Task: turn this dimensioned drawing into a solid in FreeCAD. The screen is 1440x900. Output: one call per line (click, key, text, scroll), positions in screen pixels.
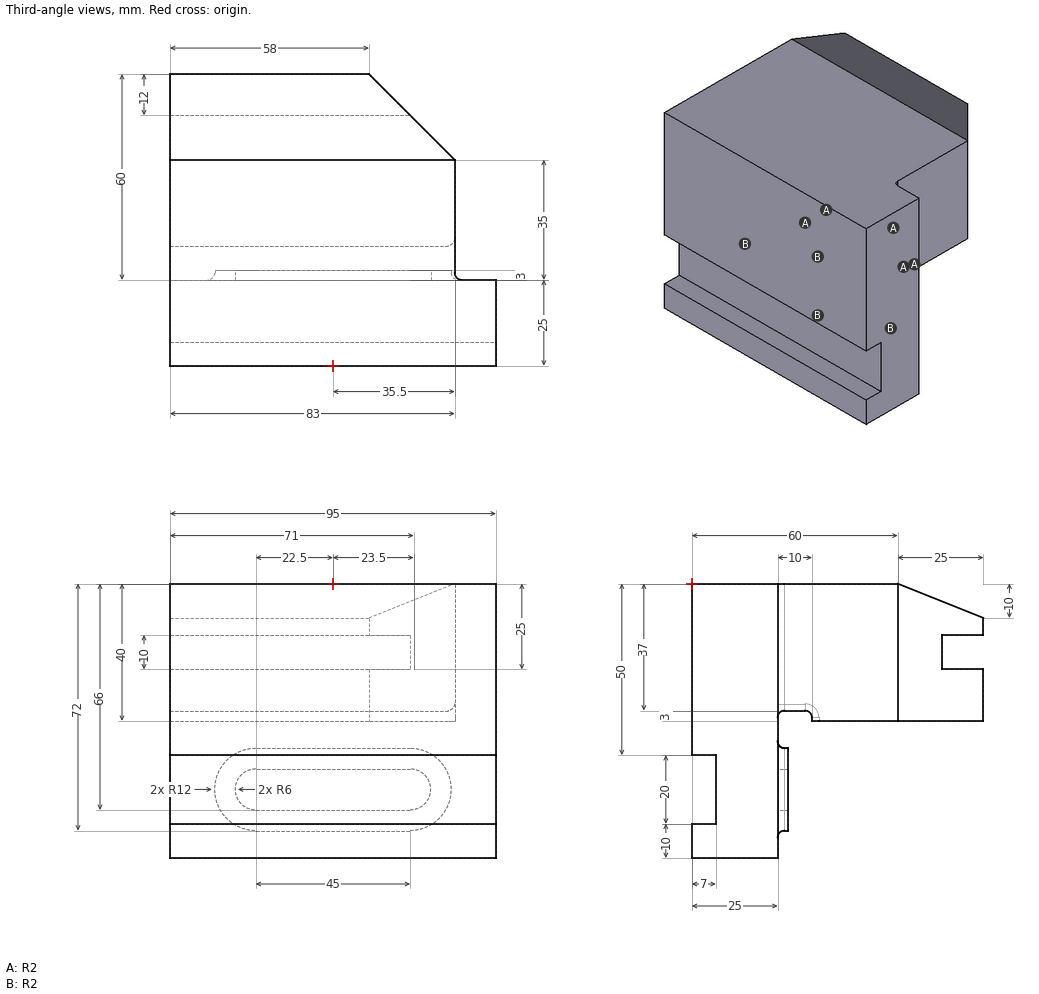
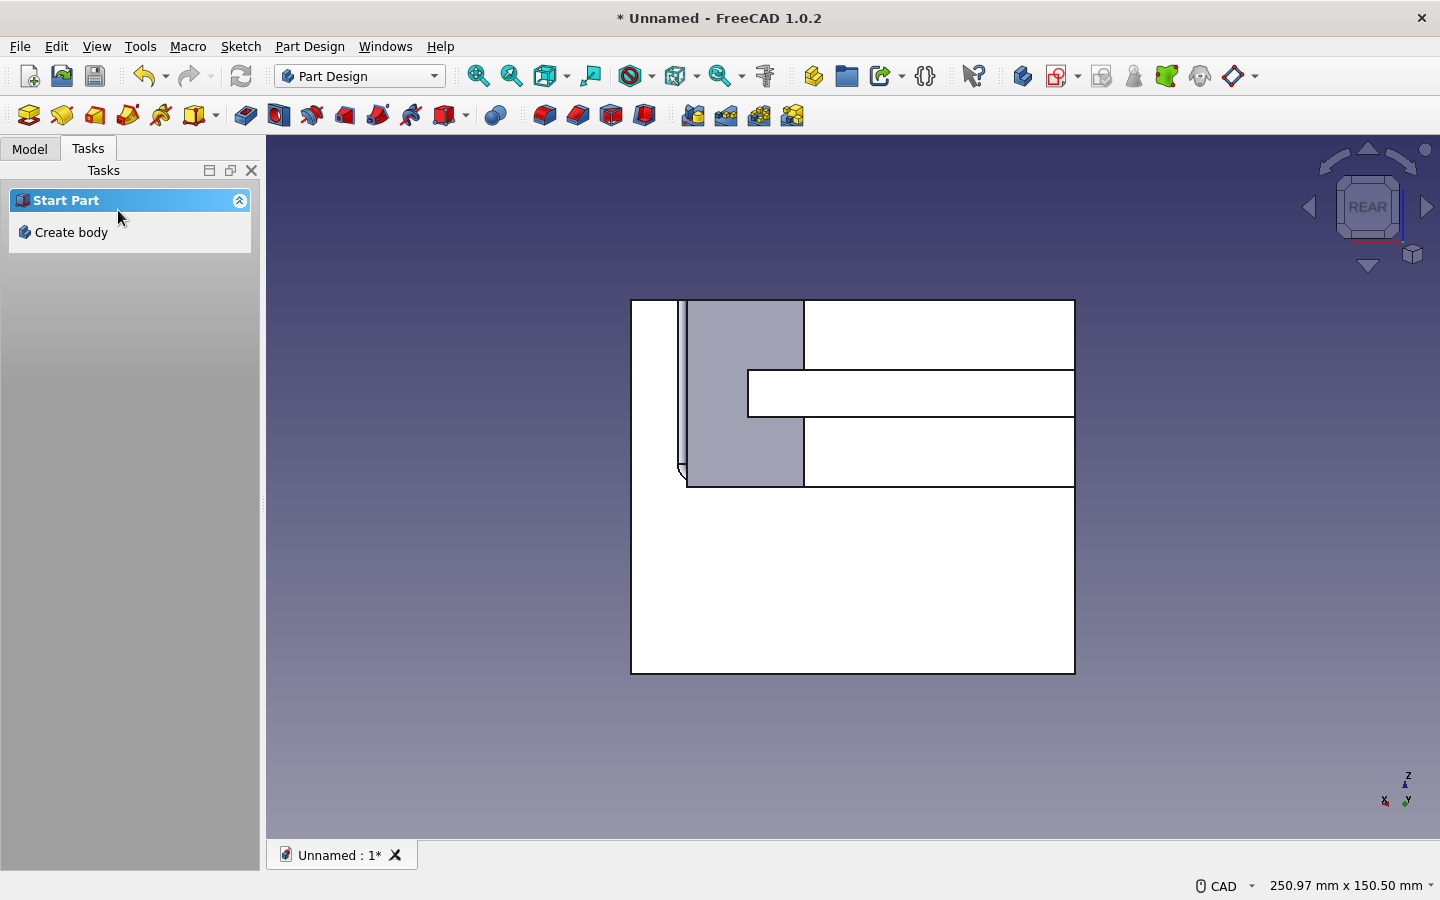
key(6)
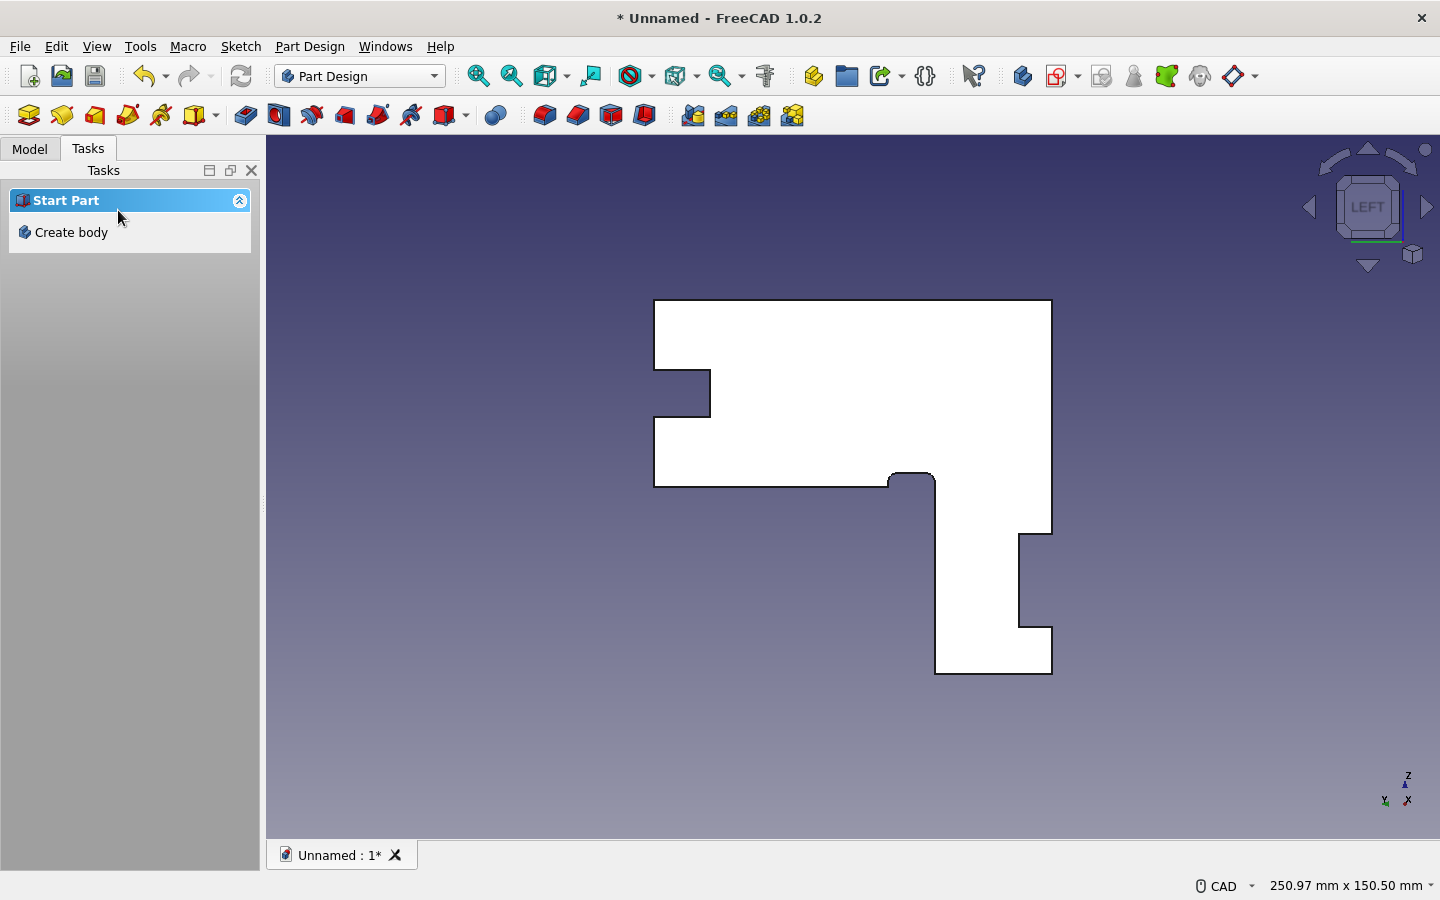
click(910, 379)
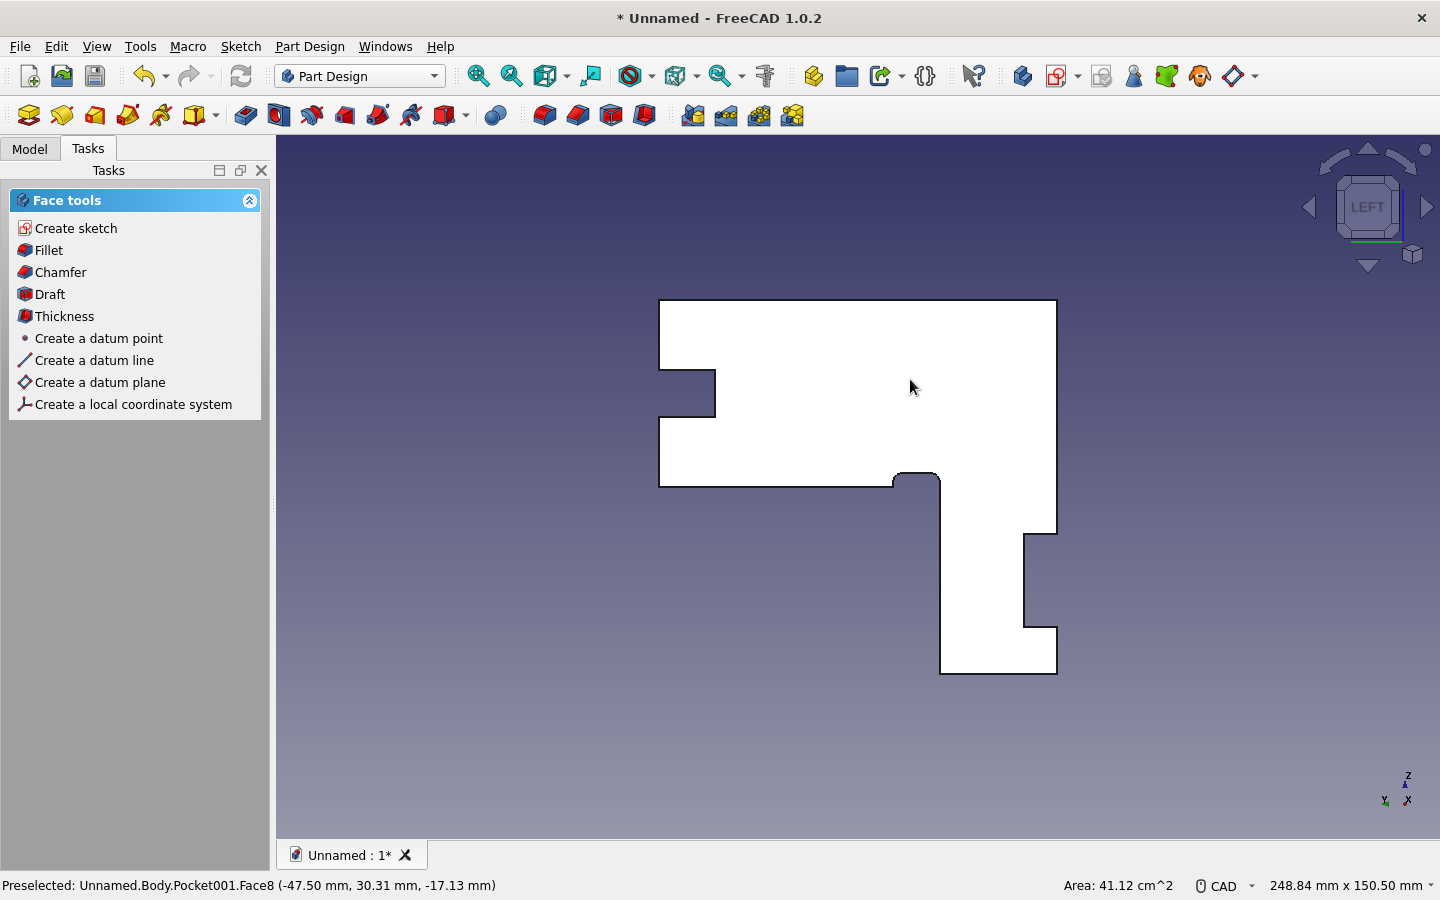
click(1056, 76)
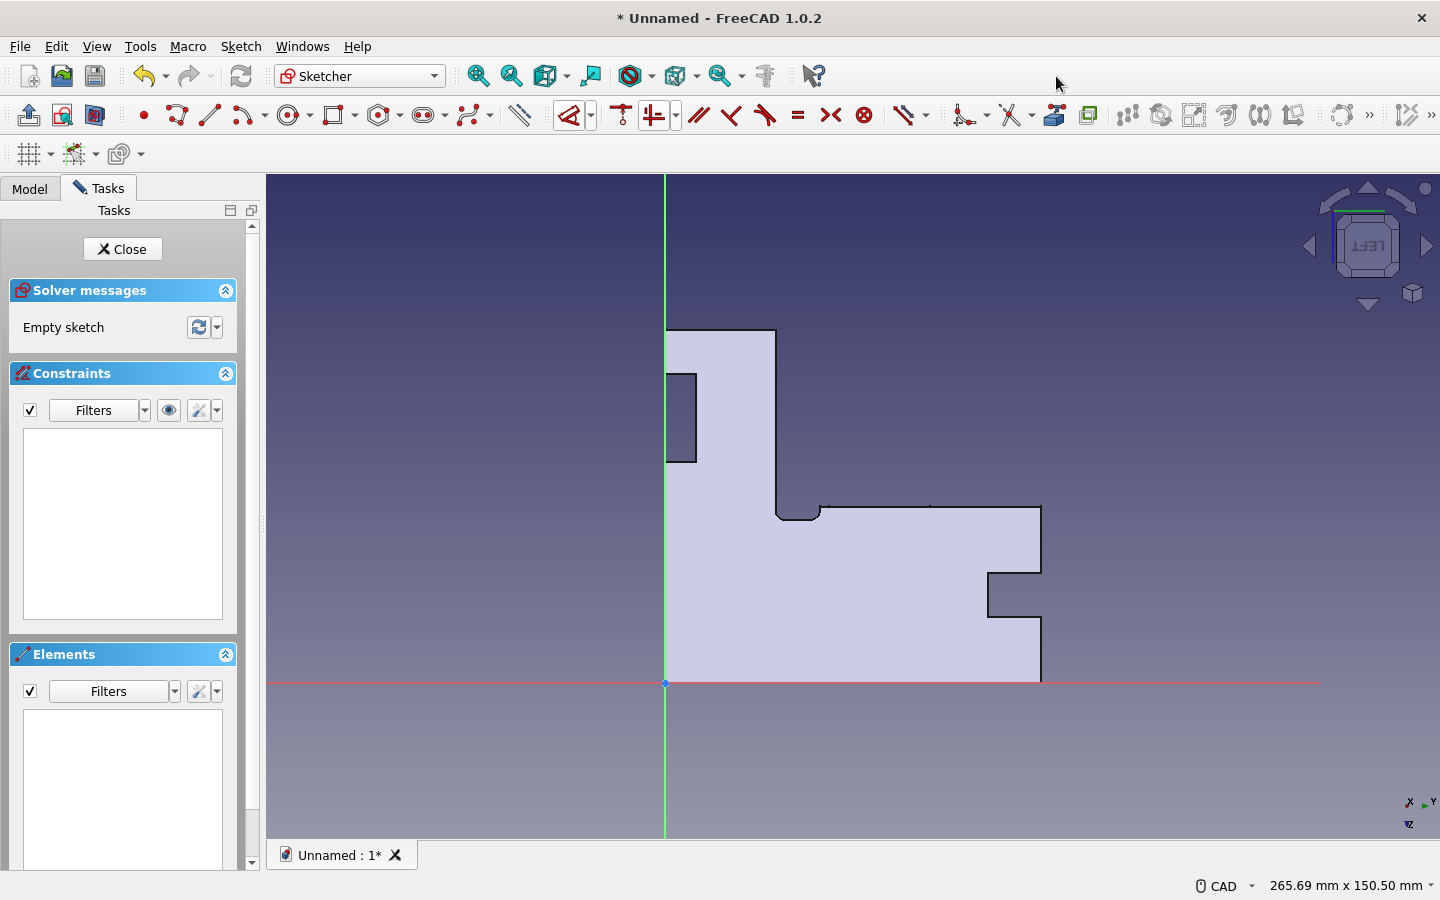
scroll(1025, 692, up, 9)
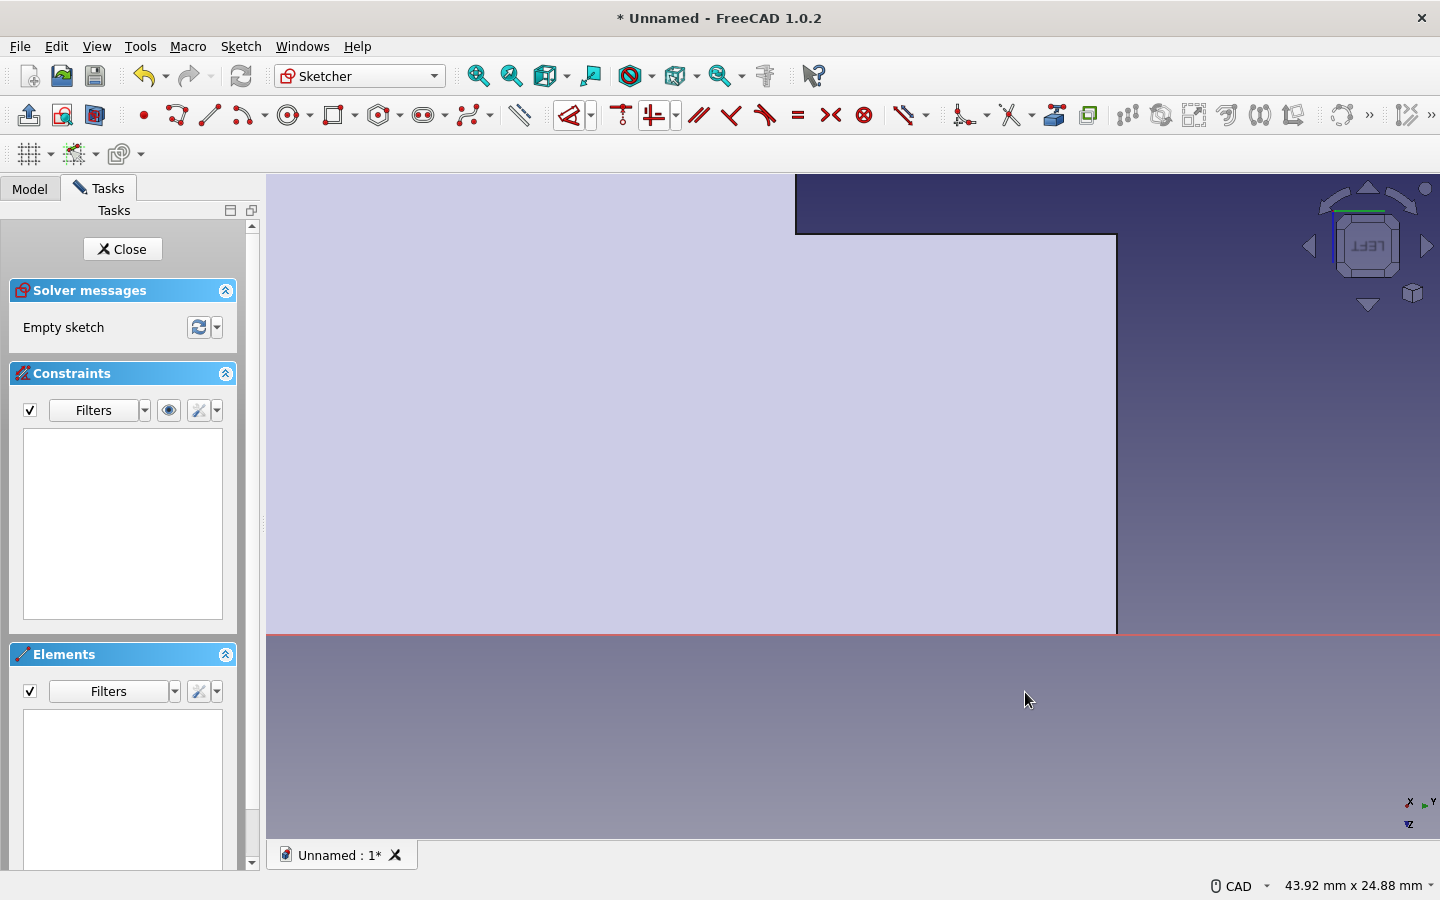
click(177, 116)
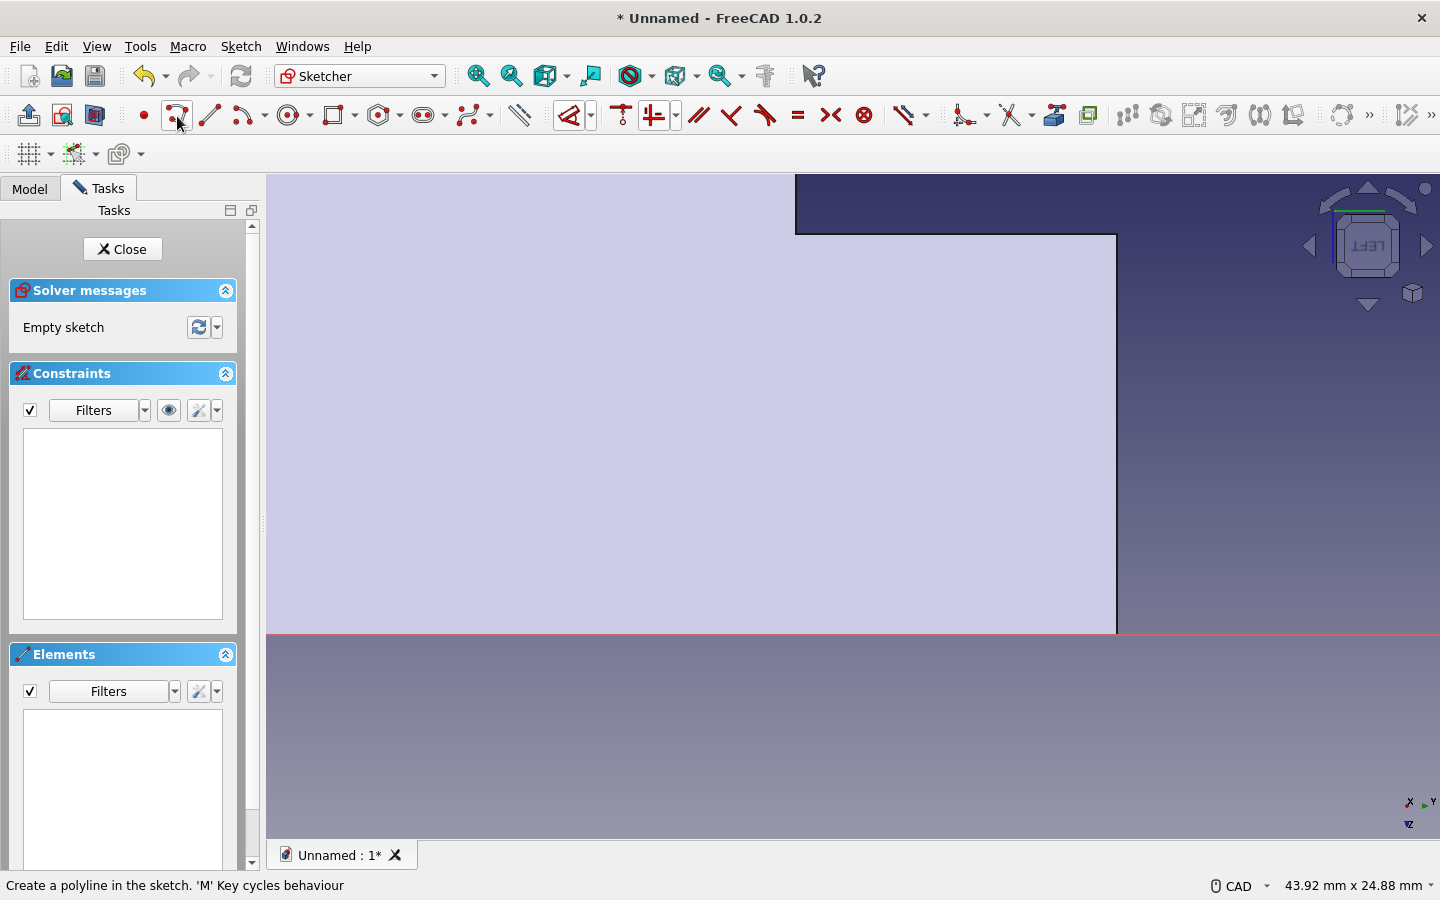
click(449, 635)
click(1117, 626)
click(1117, 368)
click(449, 635)
key(Escape)
key(Escape)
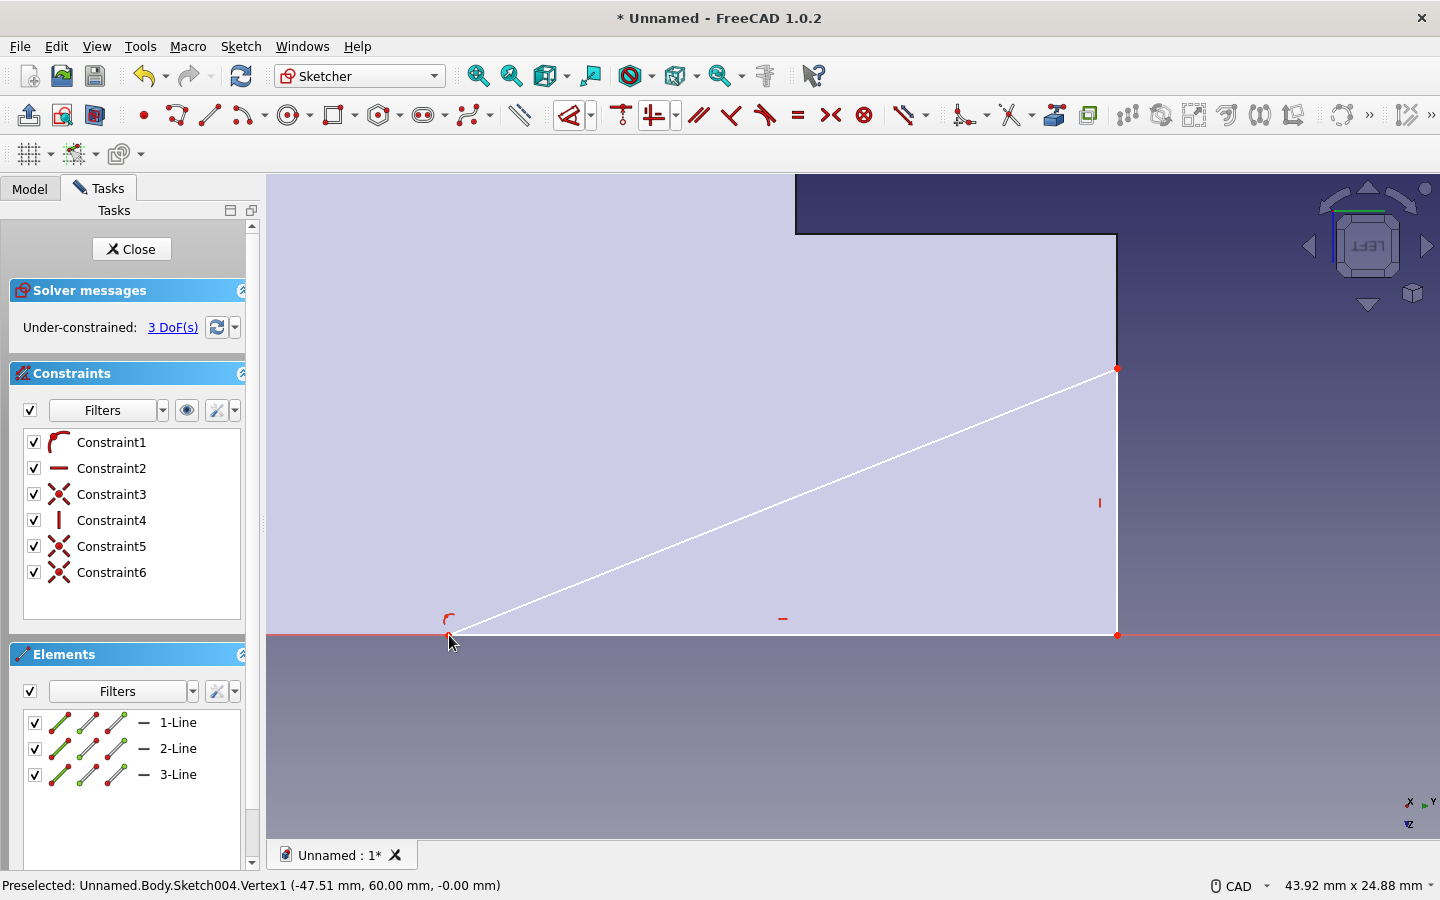
click(649, 635)